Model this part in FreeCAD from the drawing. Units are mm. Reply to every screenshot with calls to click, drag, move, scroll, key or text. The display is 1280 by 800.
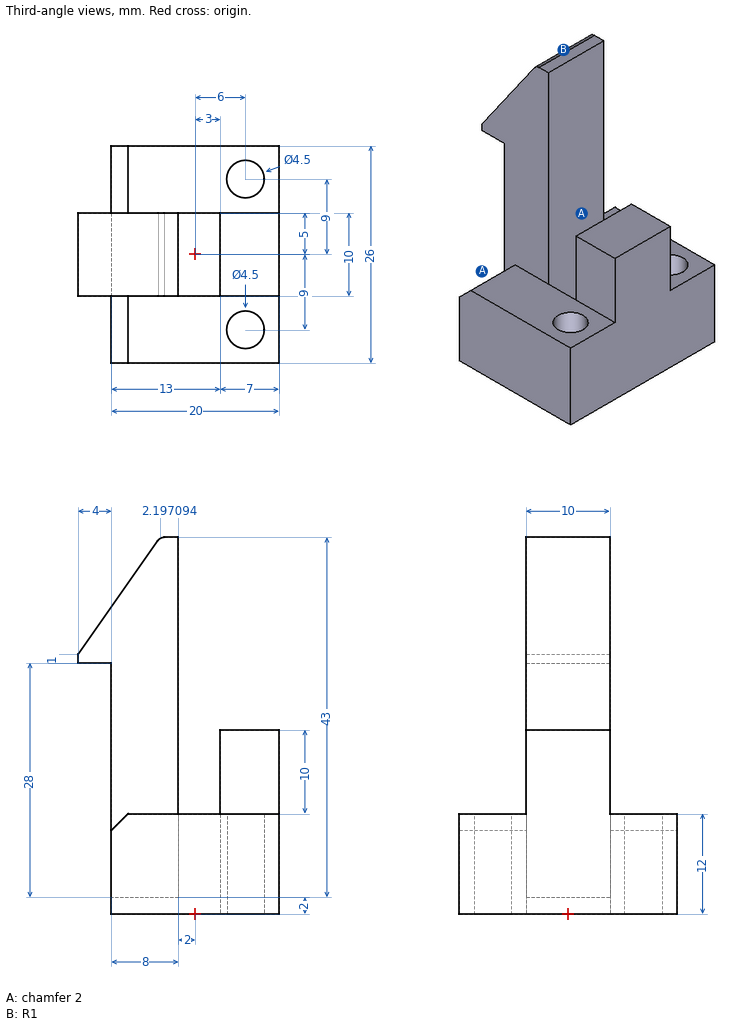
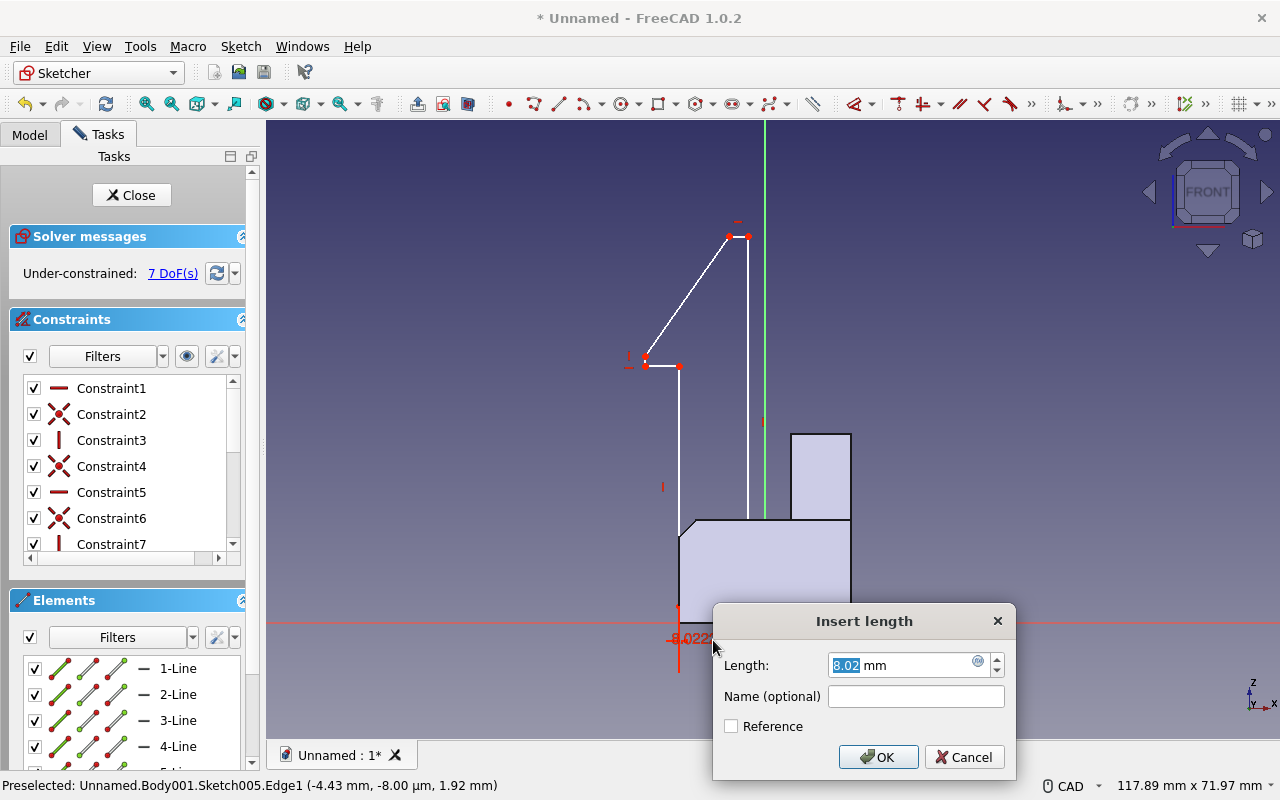
text(8)
key(Return)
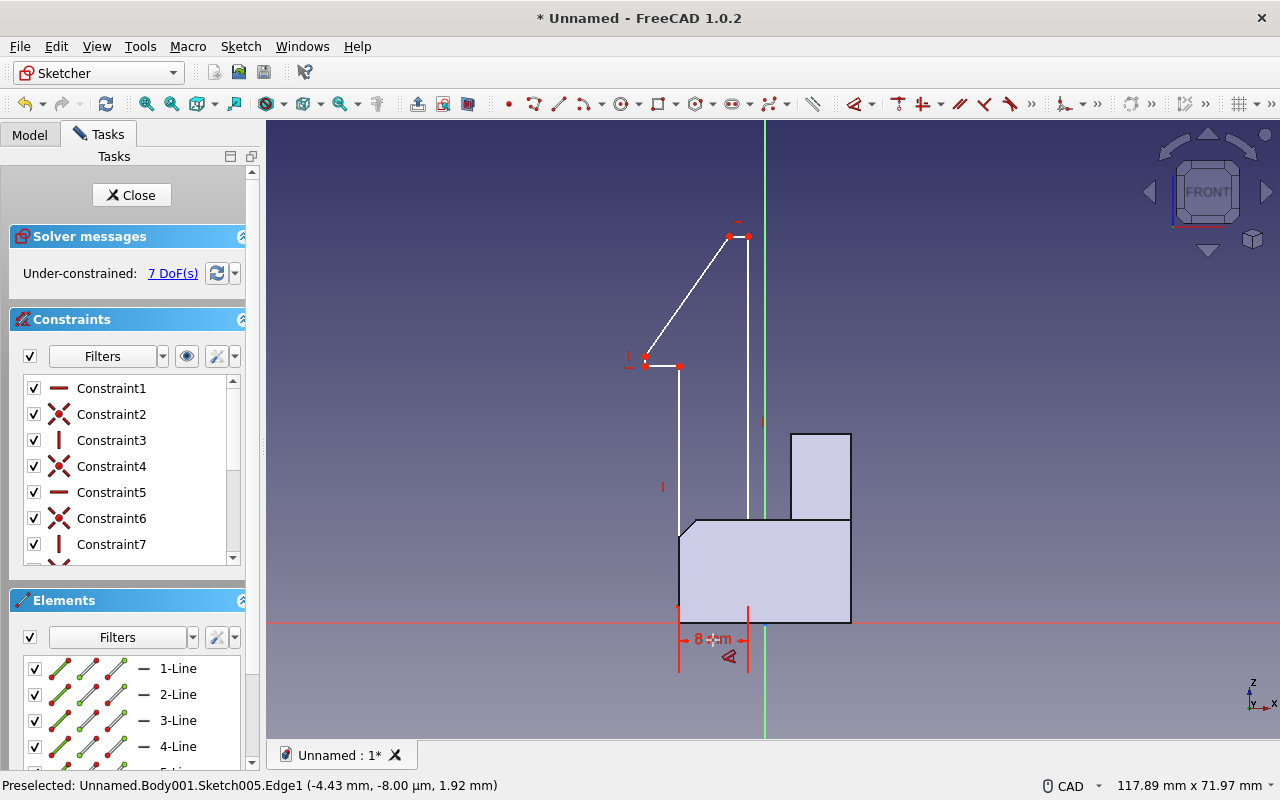
scroll(669, 366, up, 2)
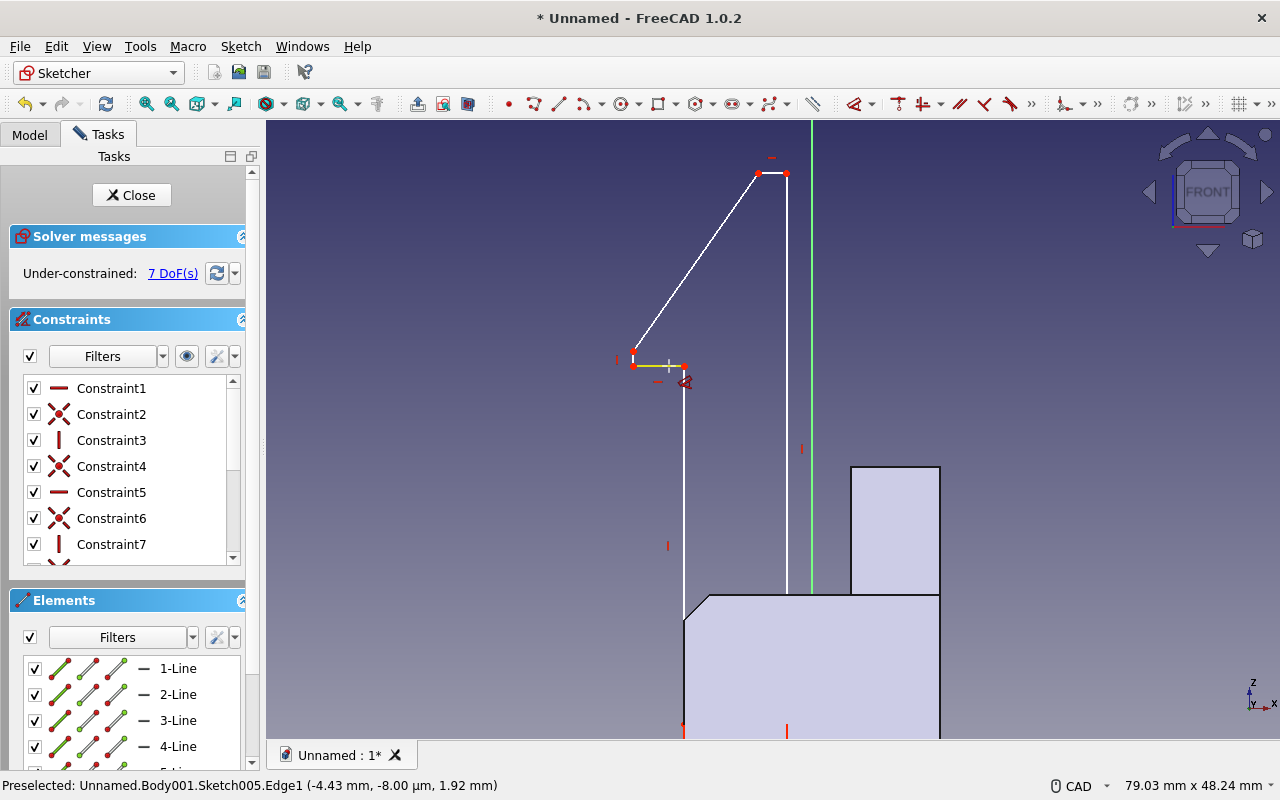
click(669, 366)
click(670, 332)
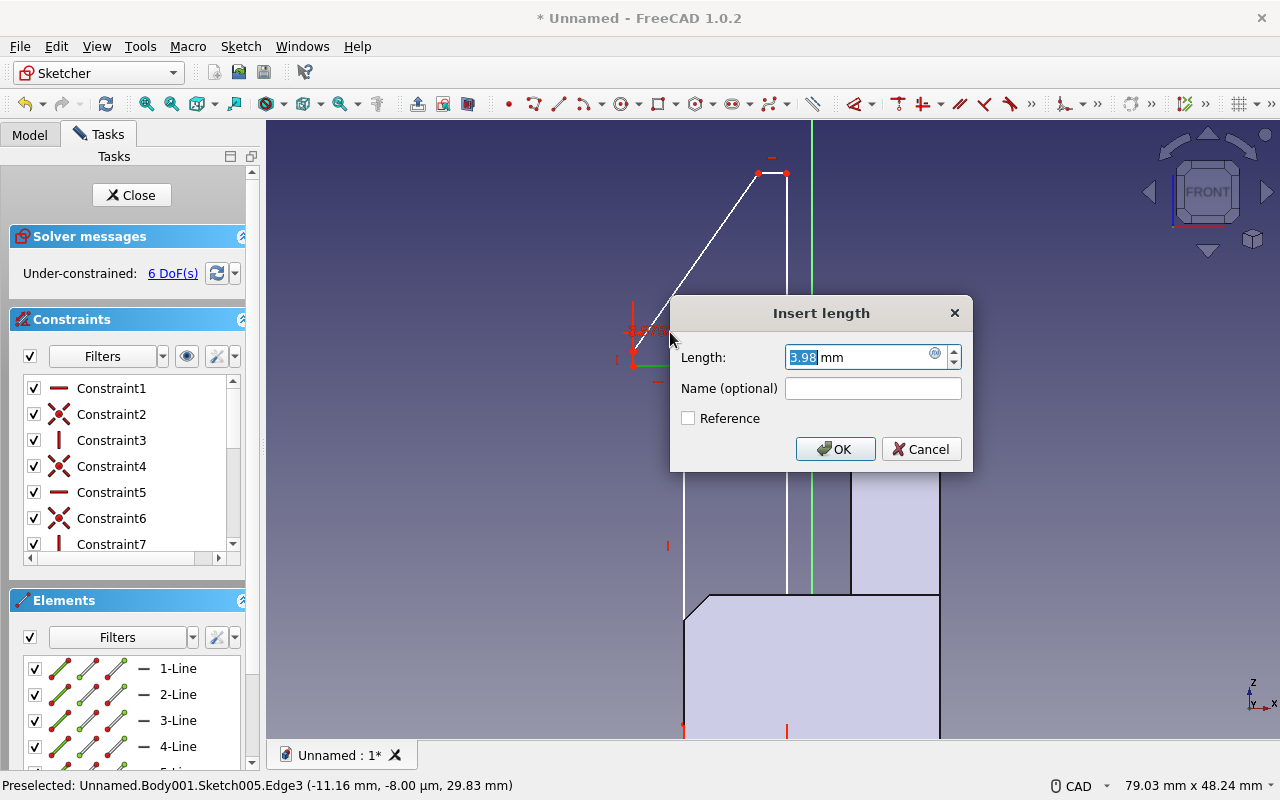
text(4)
key(Return)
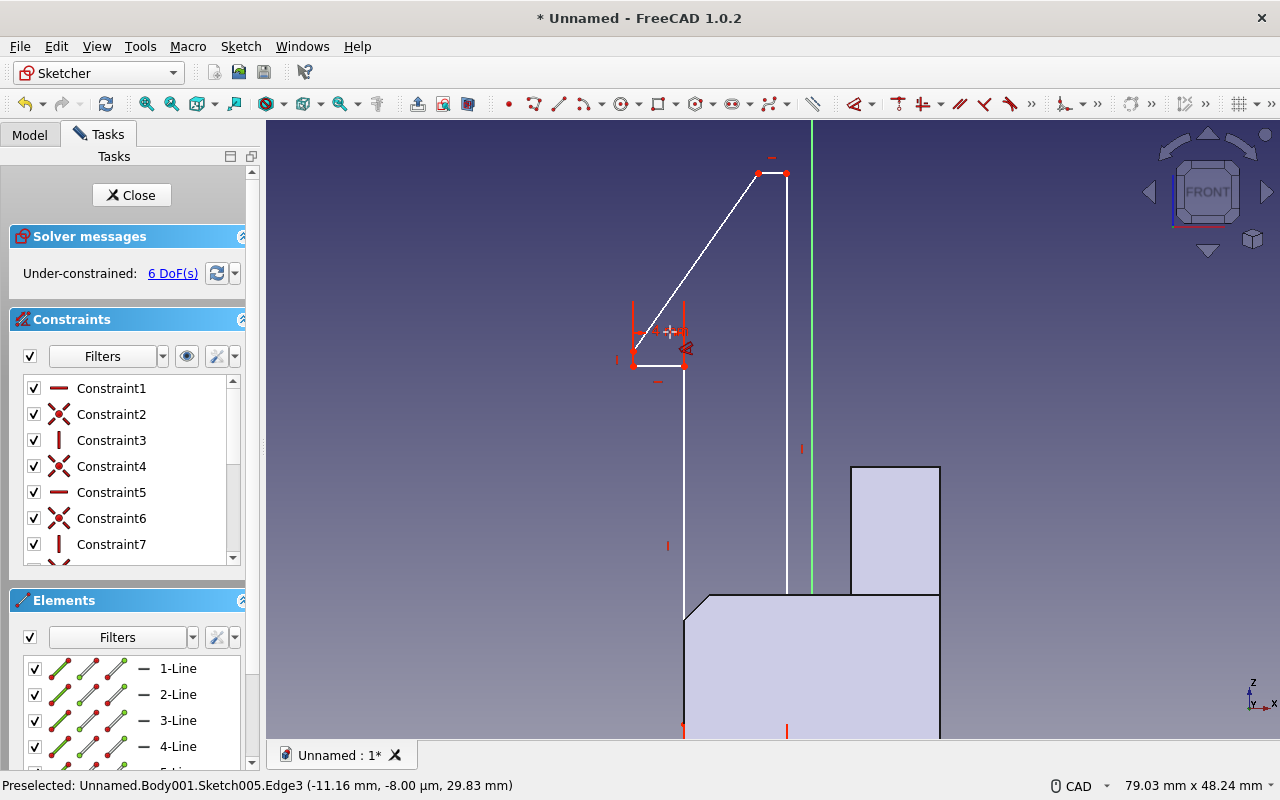
scroll(633, 359, up, 6)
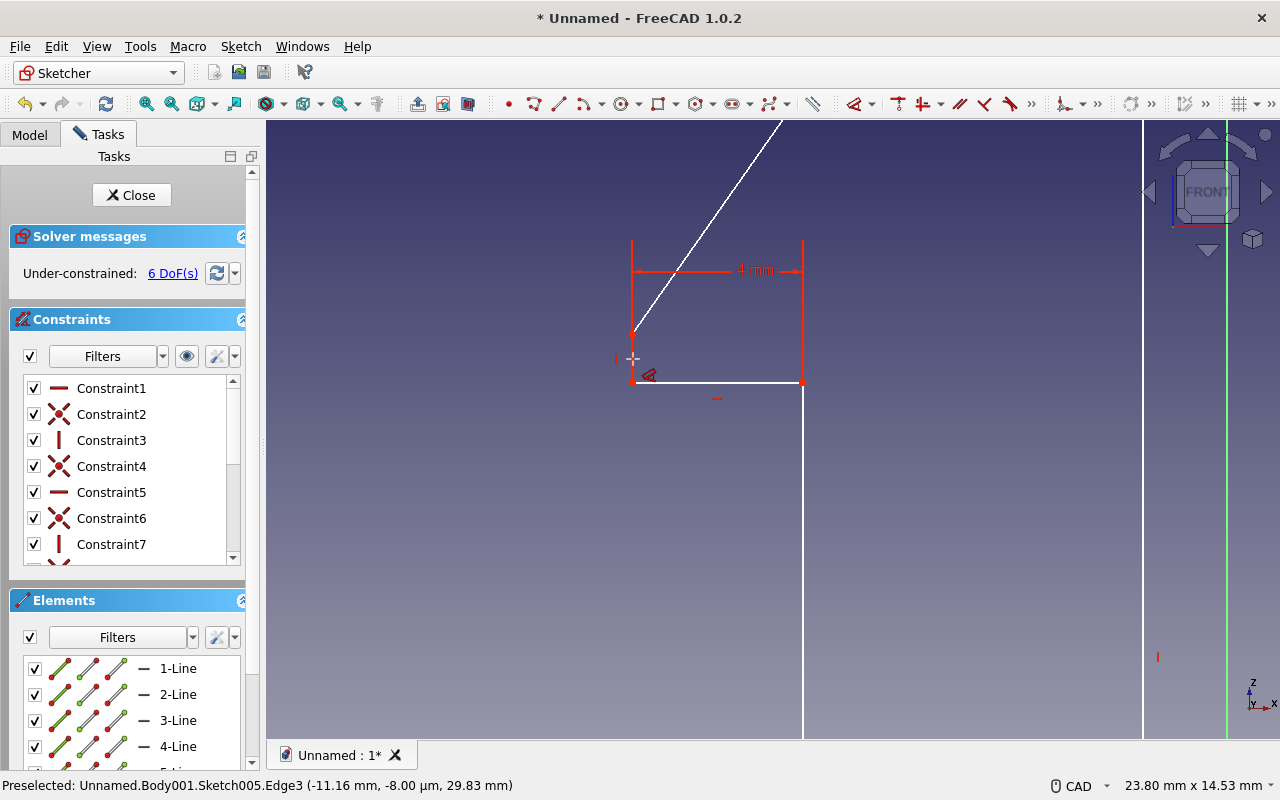
click(632, 359)
click(598, 359)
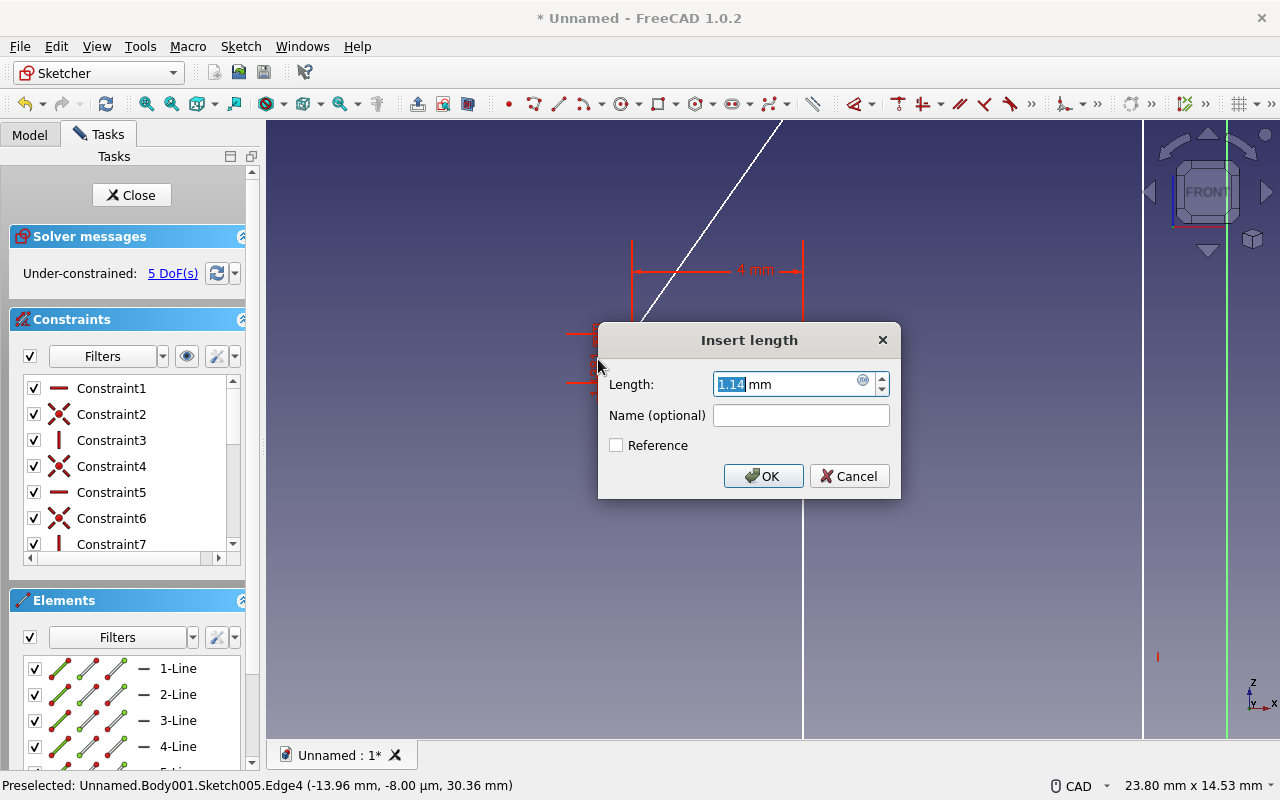
text(1)
key(Return)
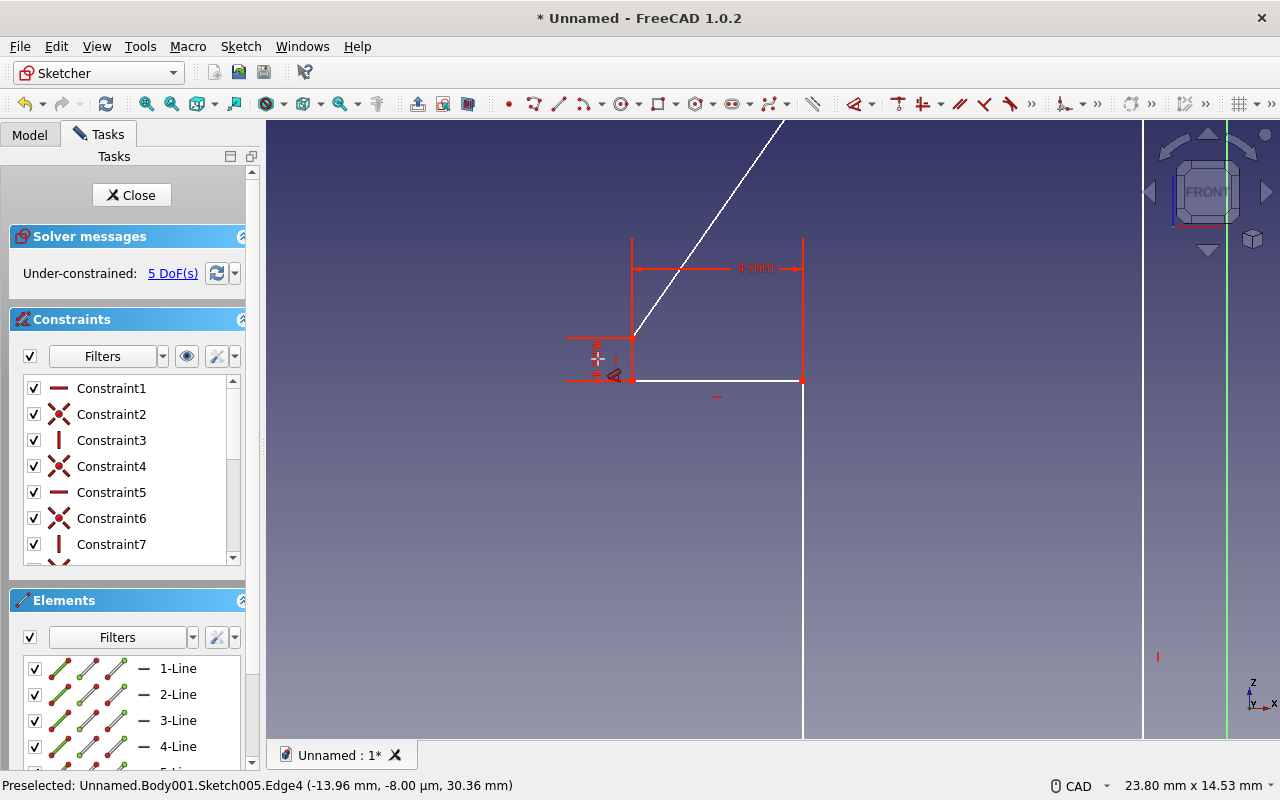
scroll(648, 362, down, 8)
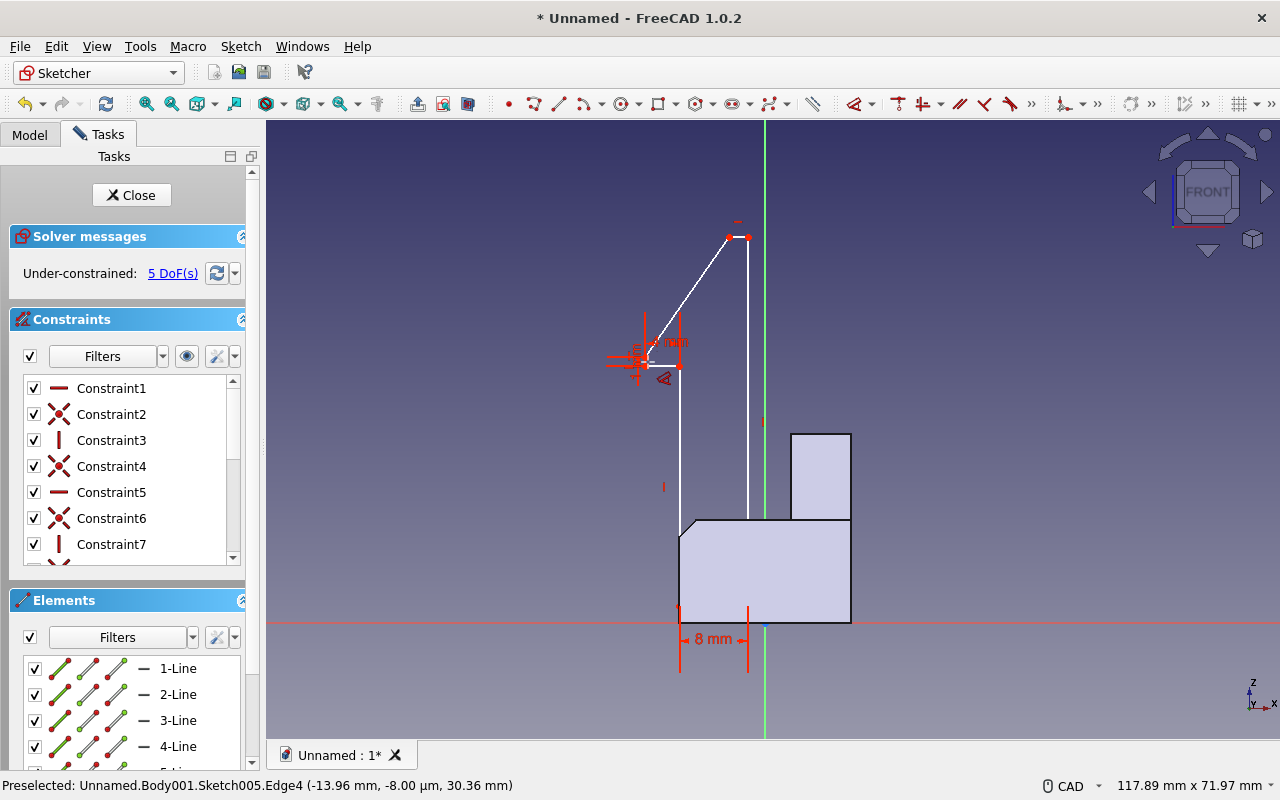
click(680, 414)
click(646, 486)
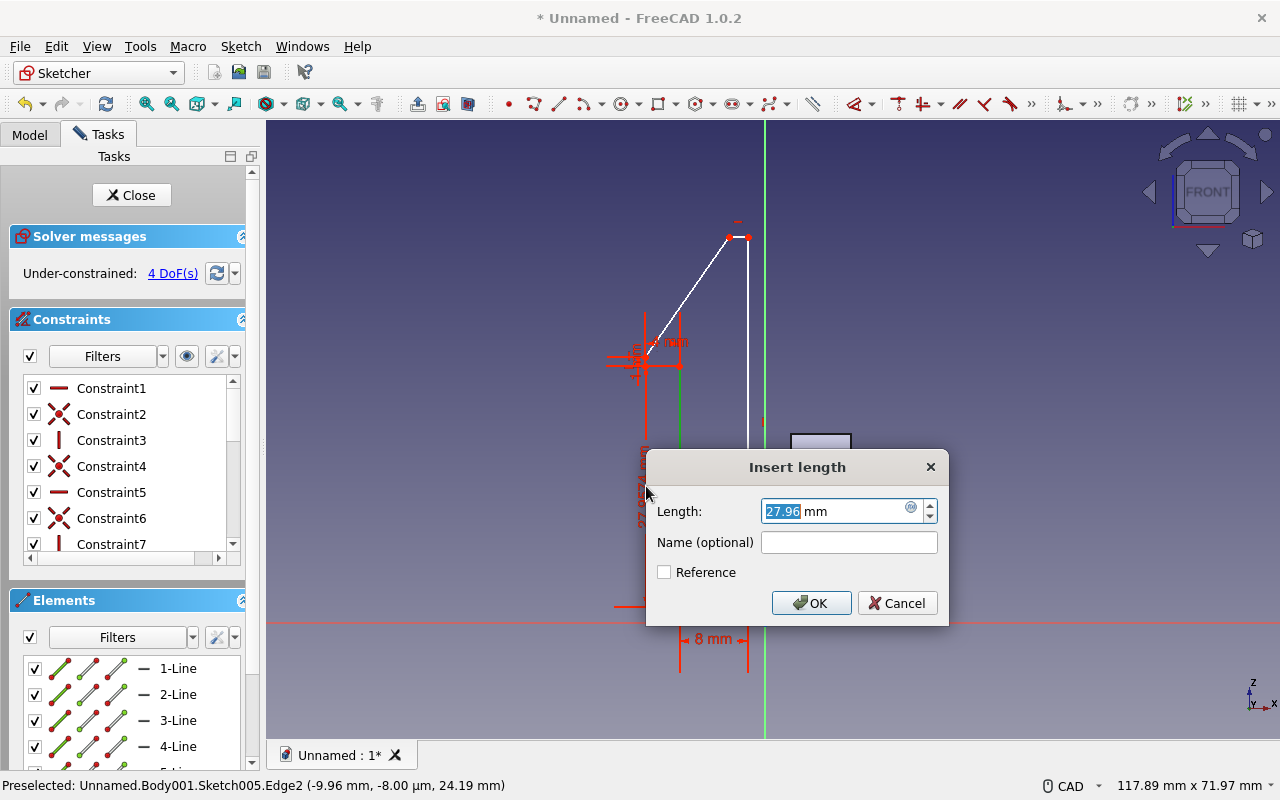
text(28)
key(Return)